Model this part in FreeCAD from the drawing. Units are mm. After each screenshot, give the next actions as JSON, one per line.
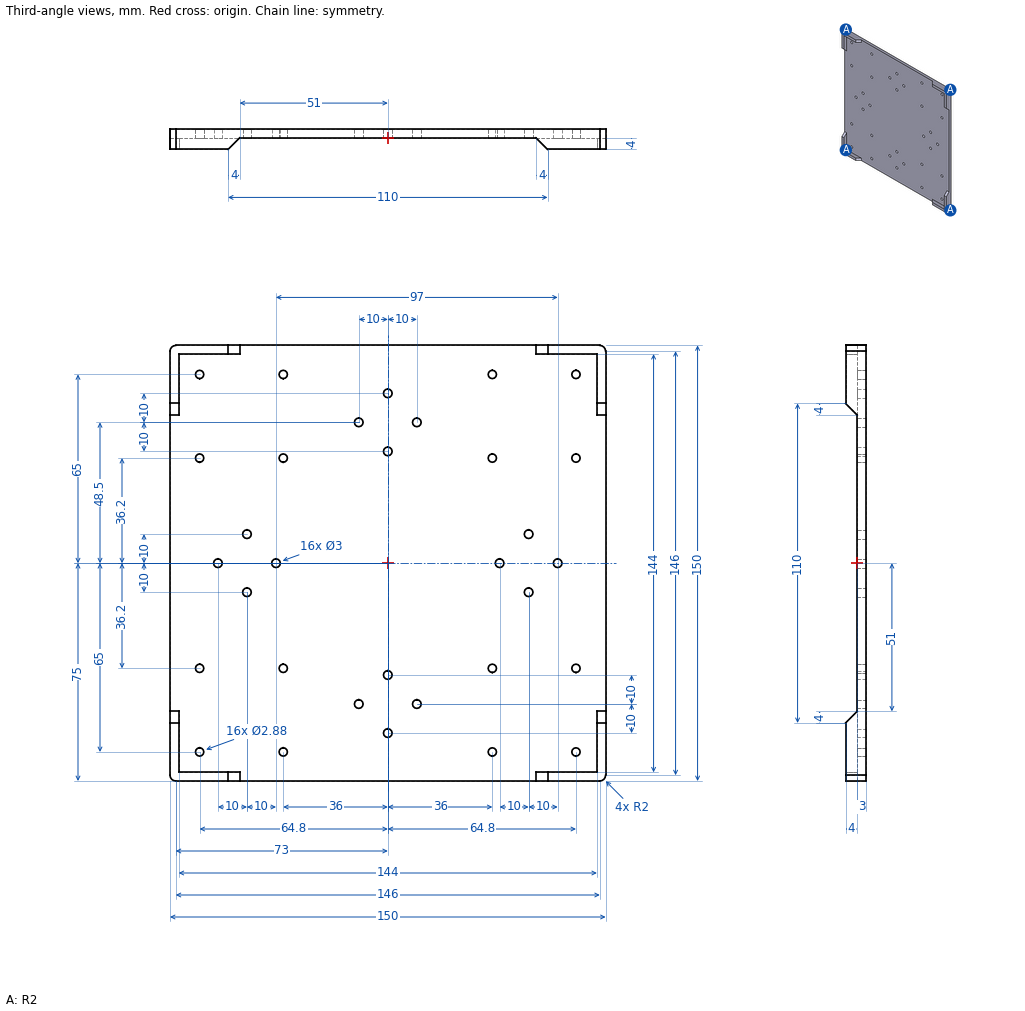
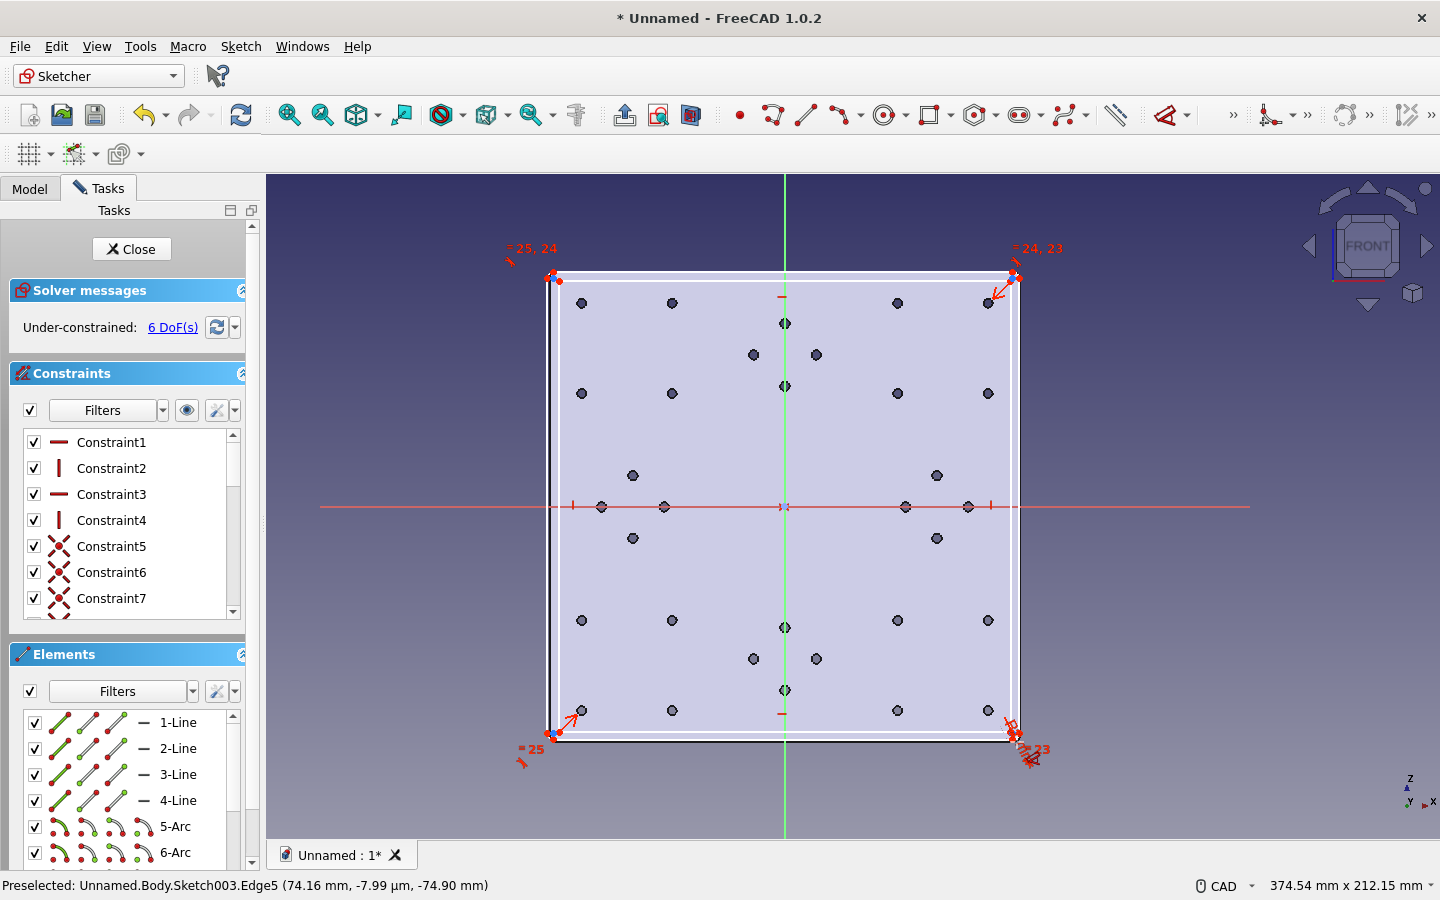
{"action": "scroll", "coordinate": [921, 740], "scroll_direction": "up", "scroll_amount": 4}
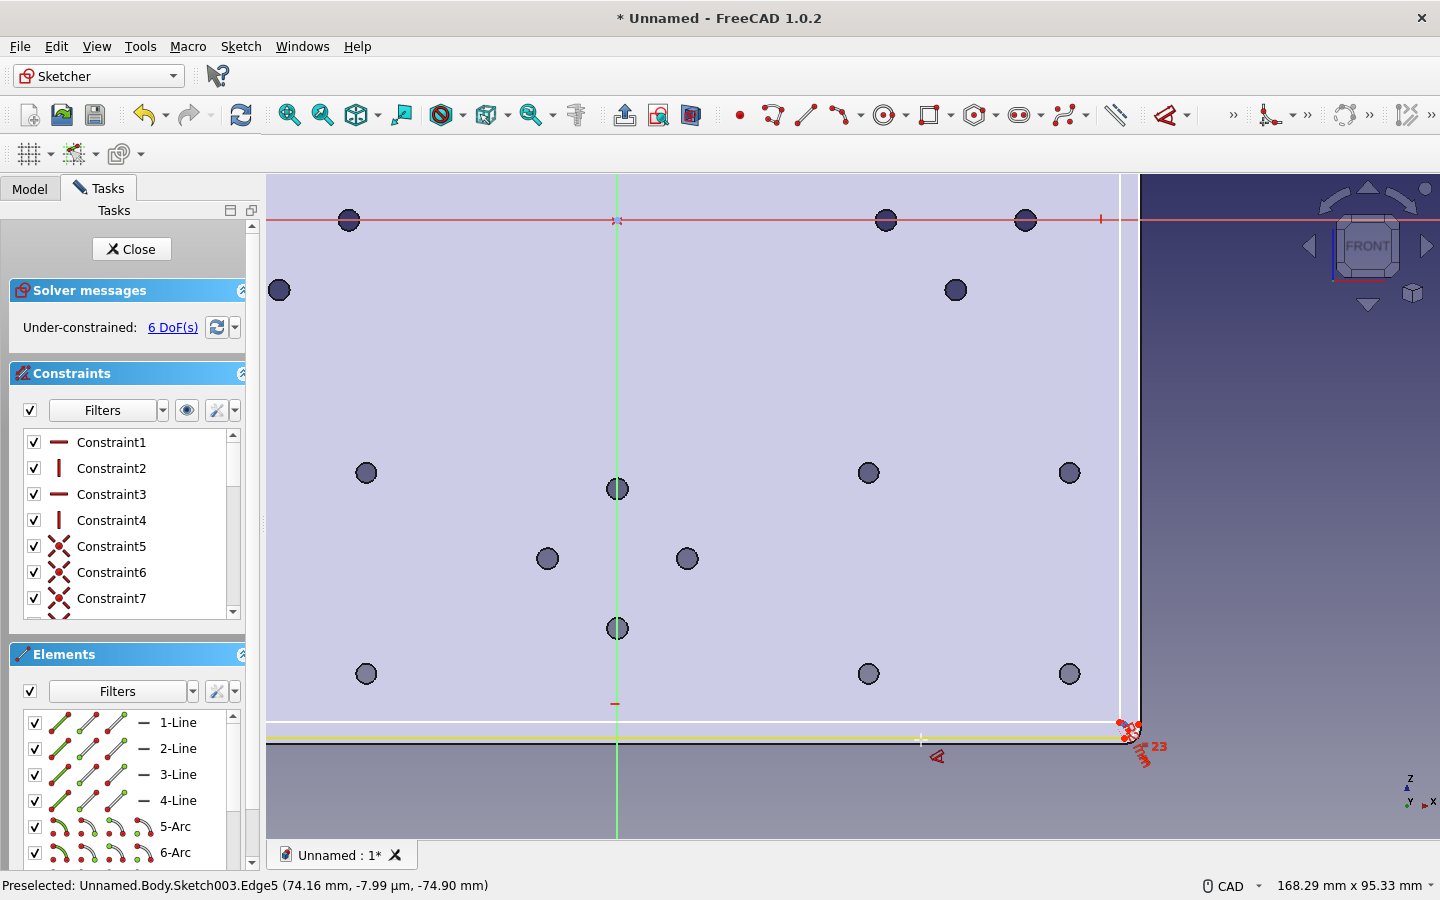
{"action": "left_click", "coordinate": [920, 738]}
{"action": "left_click", "coordinate": [709, 772]}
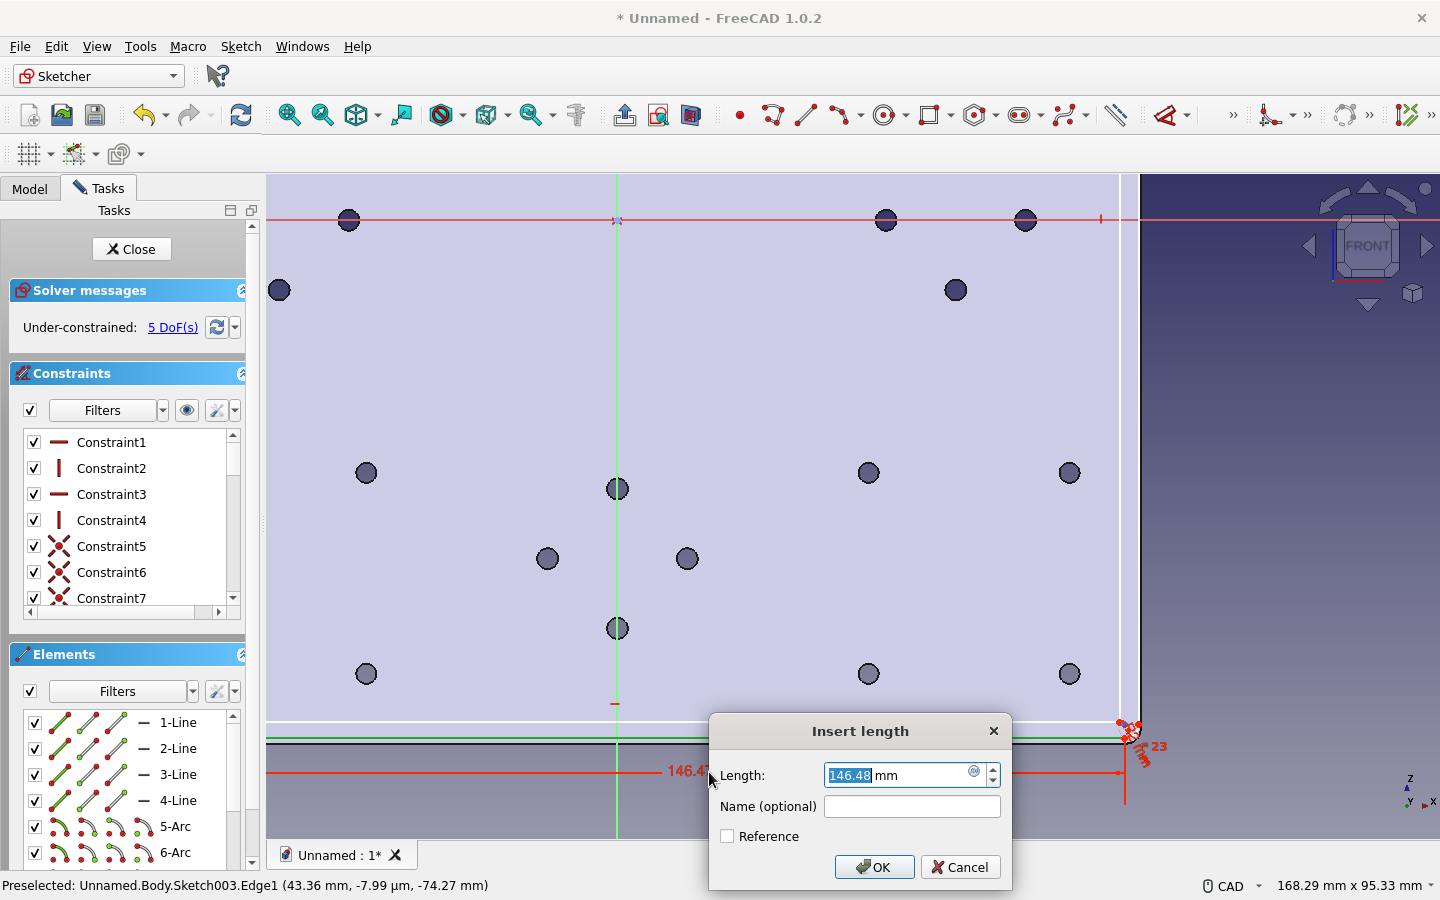
{"action": "type", "text": "146"}
{"action": "key", "text": "Return"}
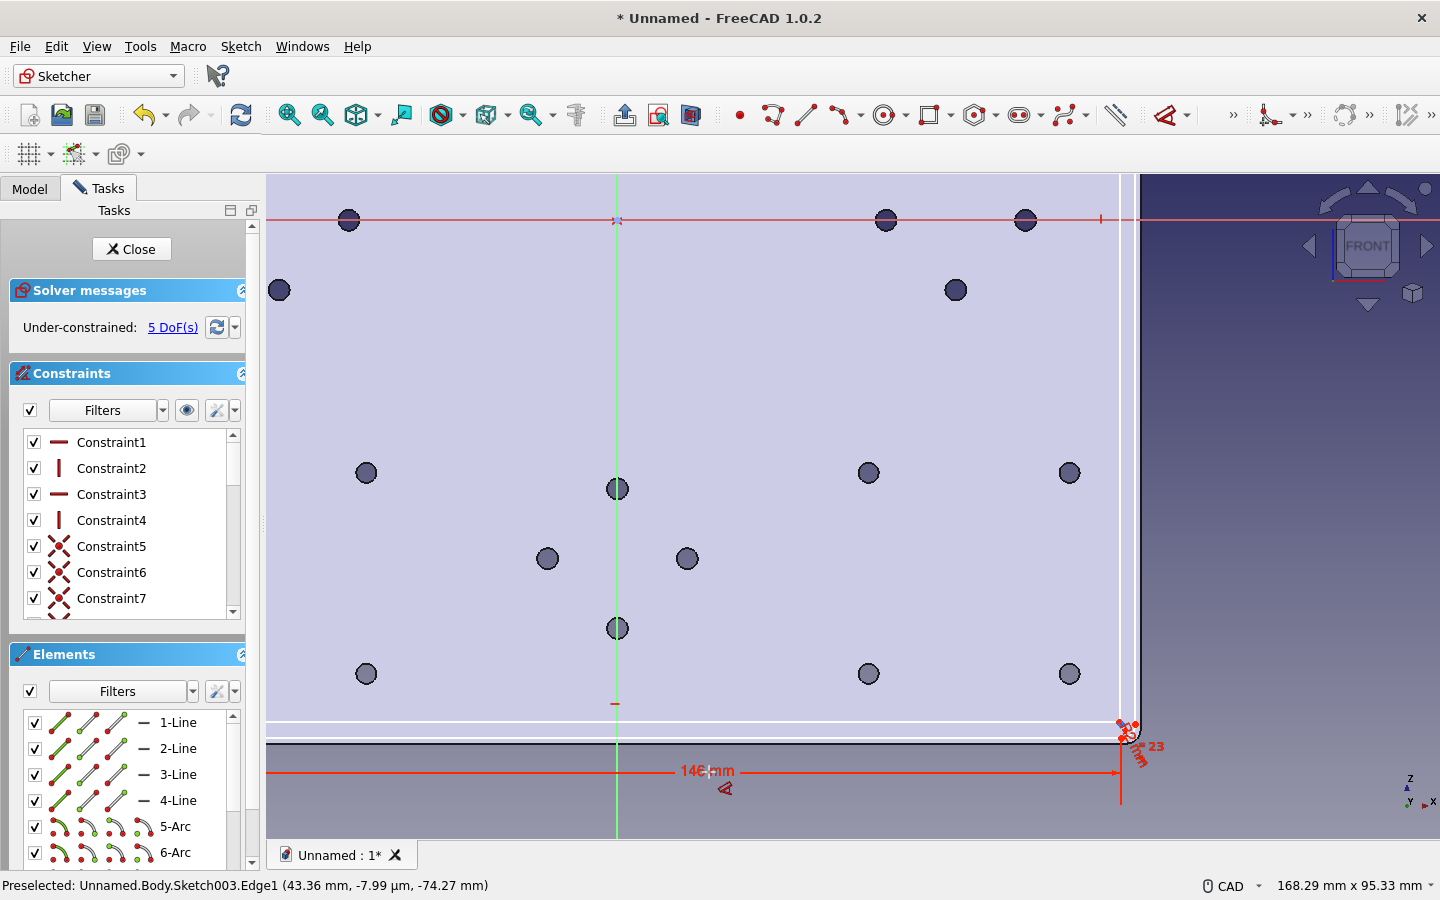
{"action": "left_click", "coordinate": [1135, 421]}
{"action": "left_click", "coordinate": [1169, 463]}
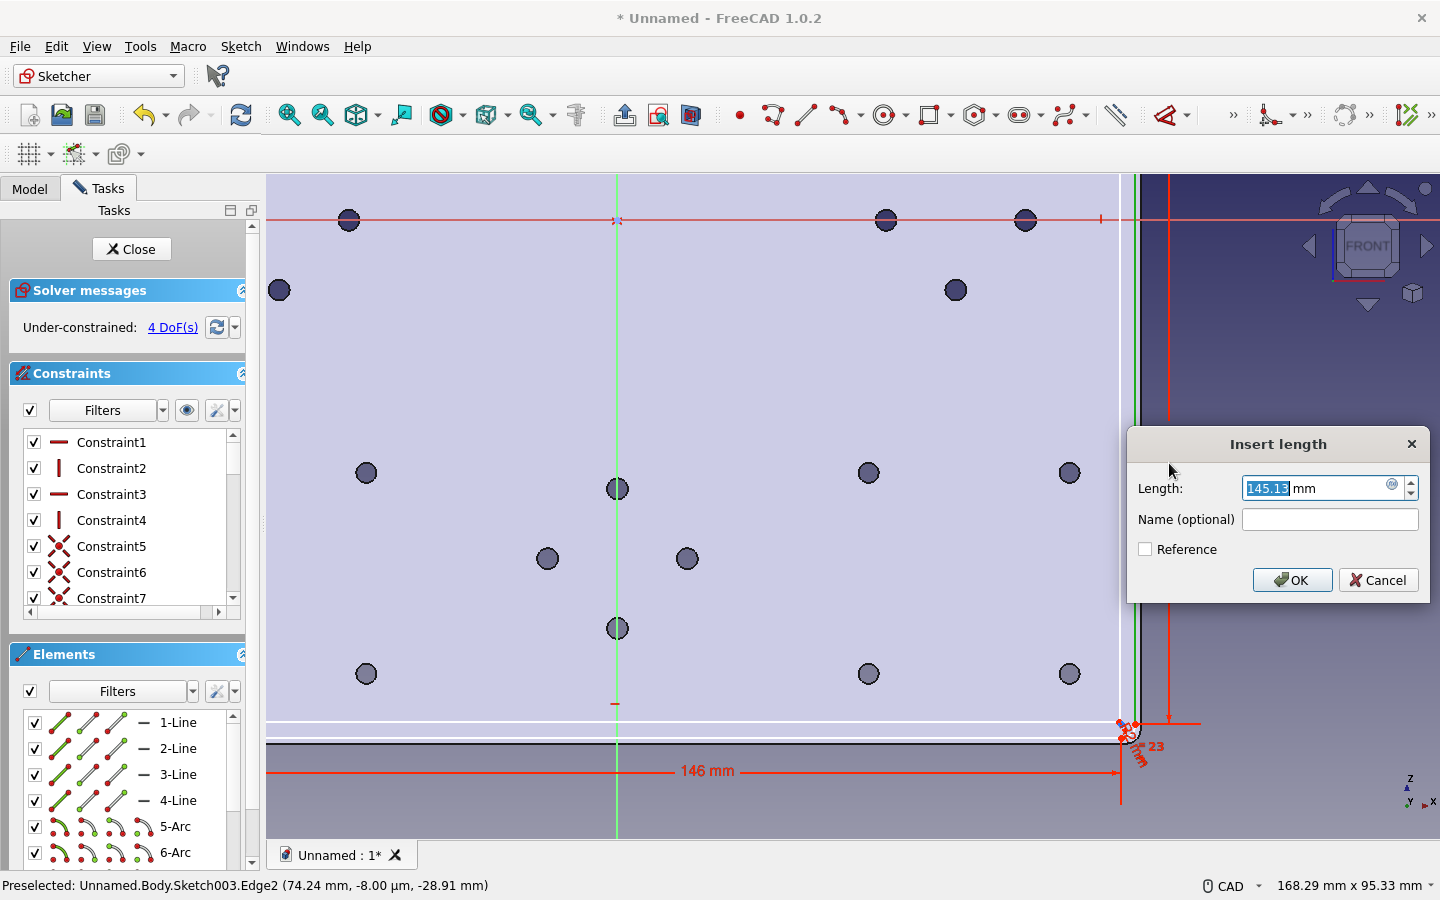
{"action": "type", "text": "146"}
{"action": "key", "text": "Return"}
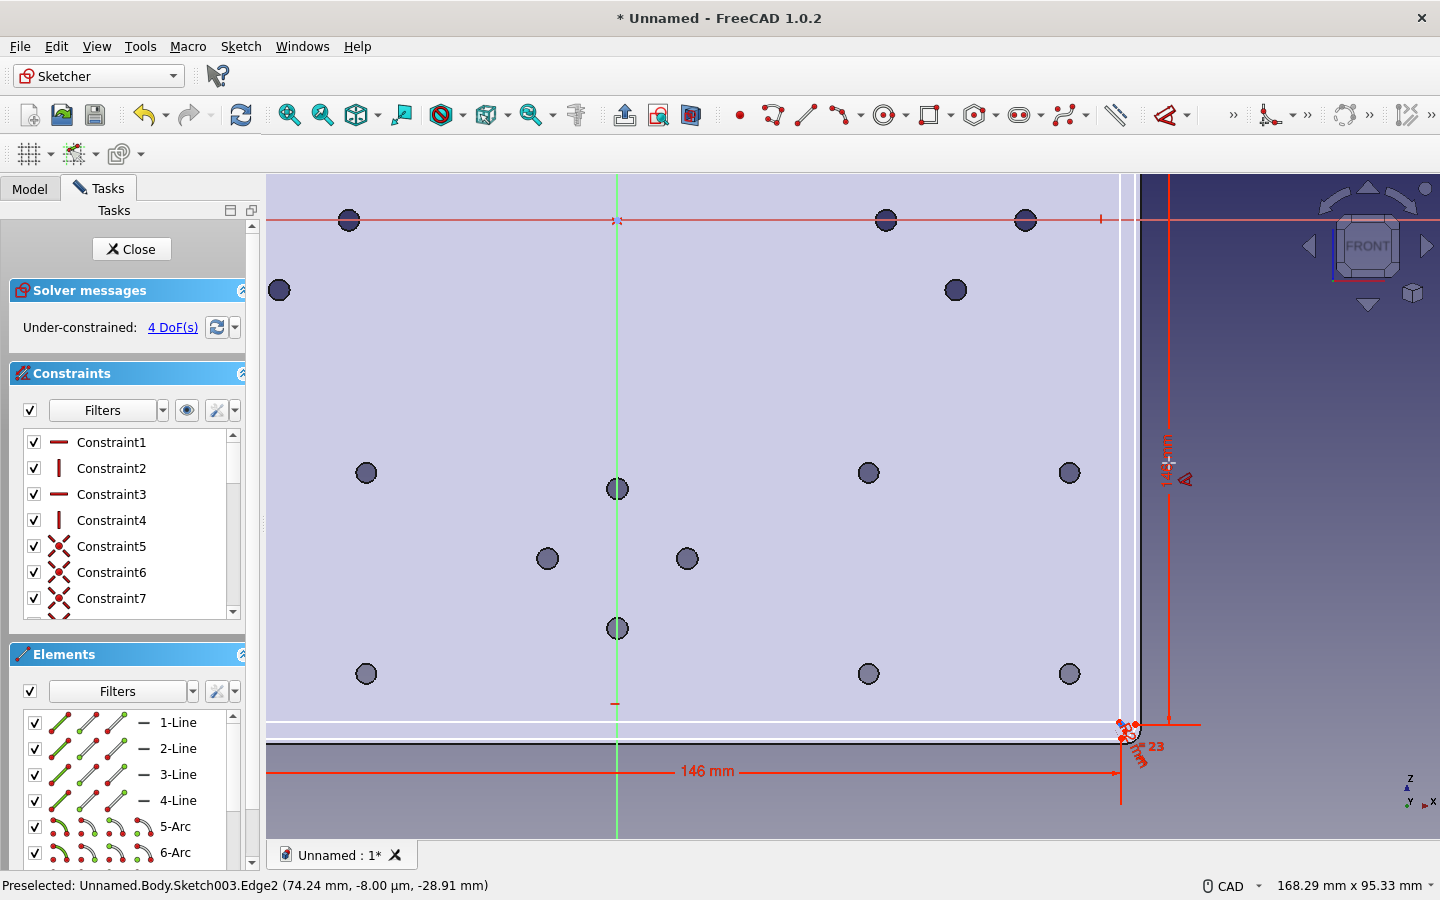
{"action": "left_click", "coordinate": [417, 722]}
{"action": "left_click", "coordinate": [517, 756]}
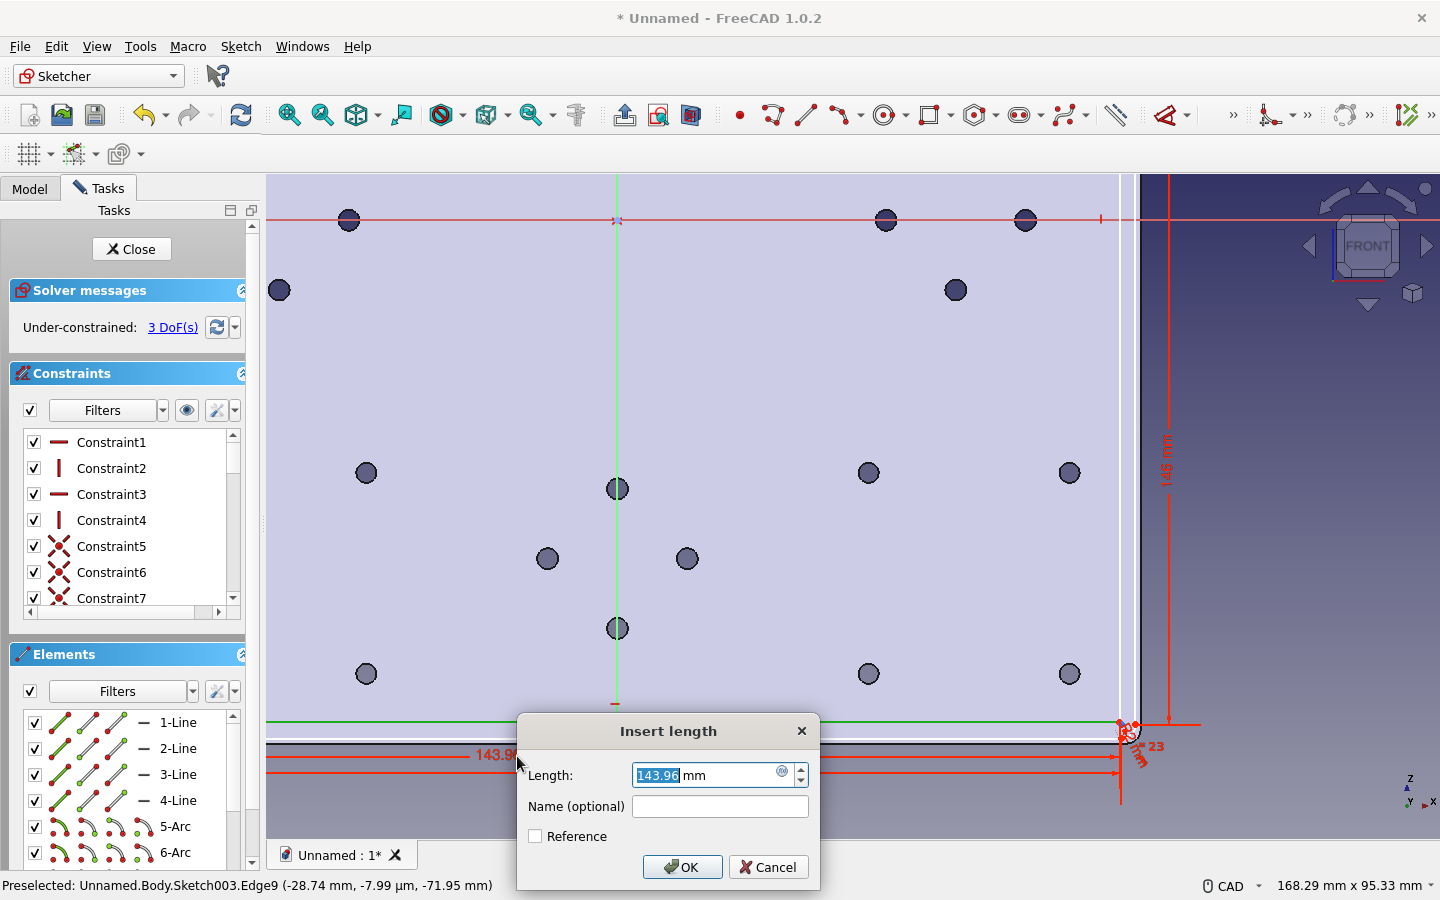
{"action": "type", "text": "144"}
{"action": "key", "text": "Return"}